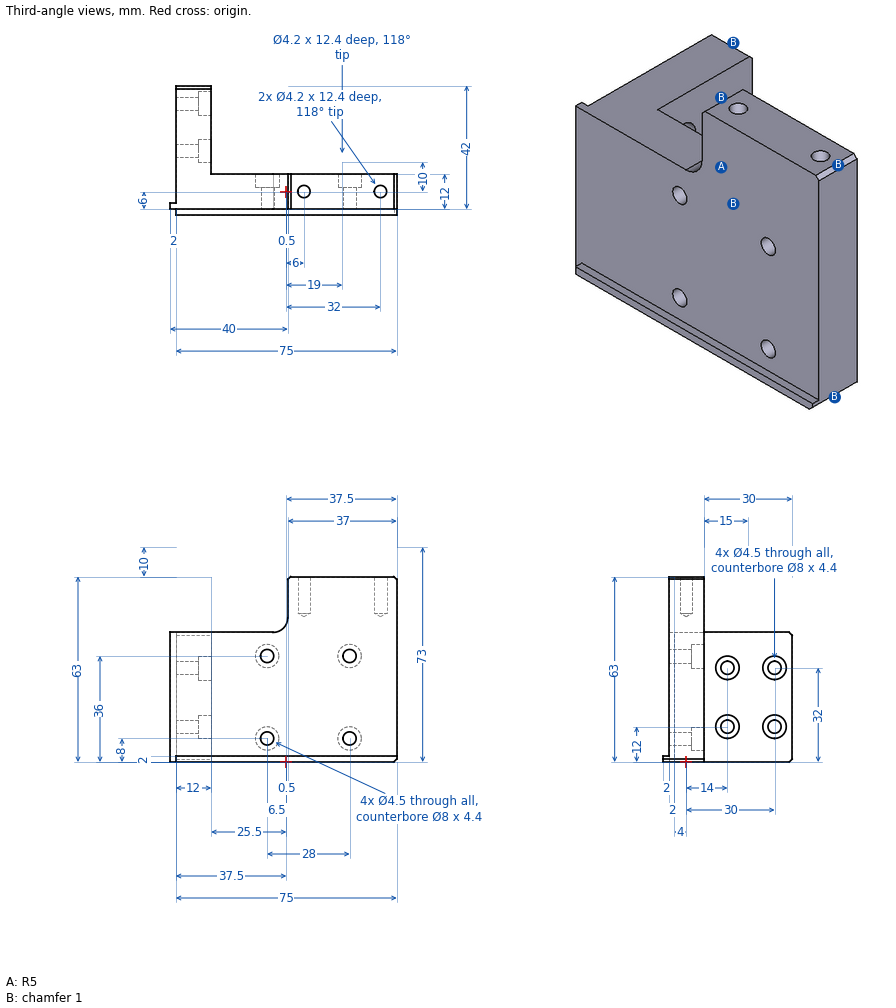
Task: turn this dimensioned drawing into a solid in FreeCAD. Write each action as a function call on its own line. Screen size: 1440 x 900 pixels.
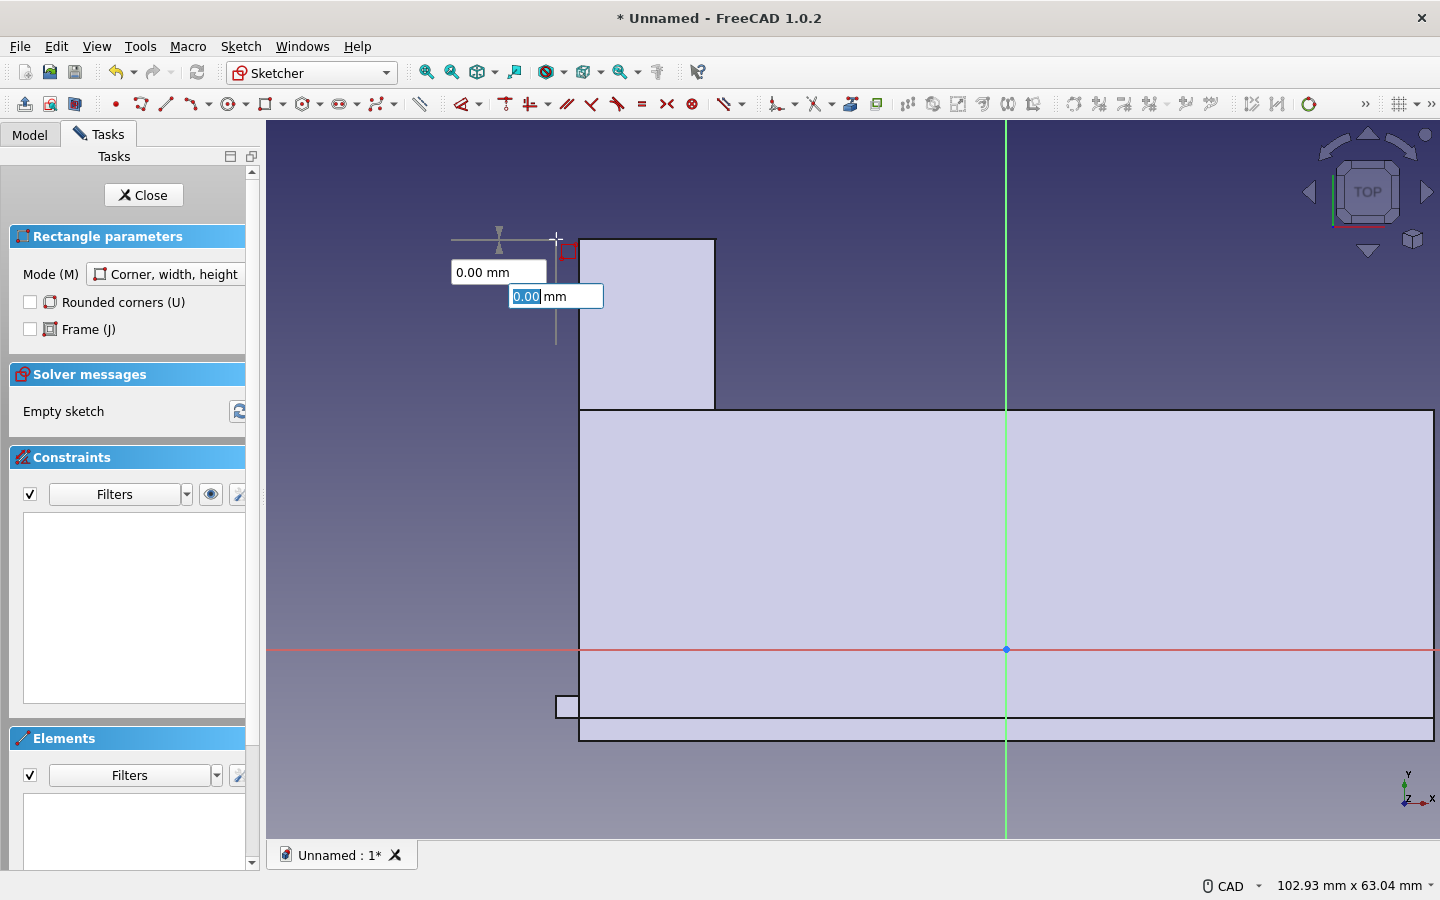
scroll(1012, 718, up, 6)
move(1011, 717)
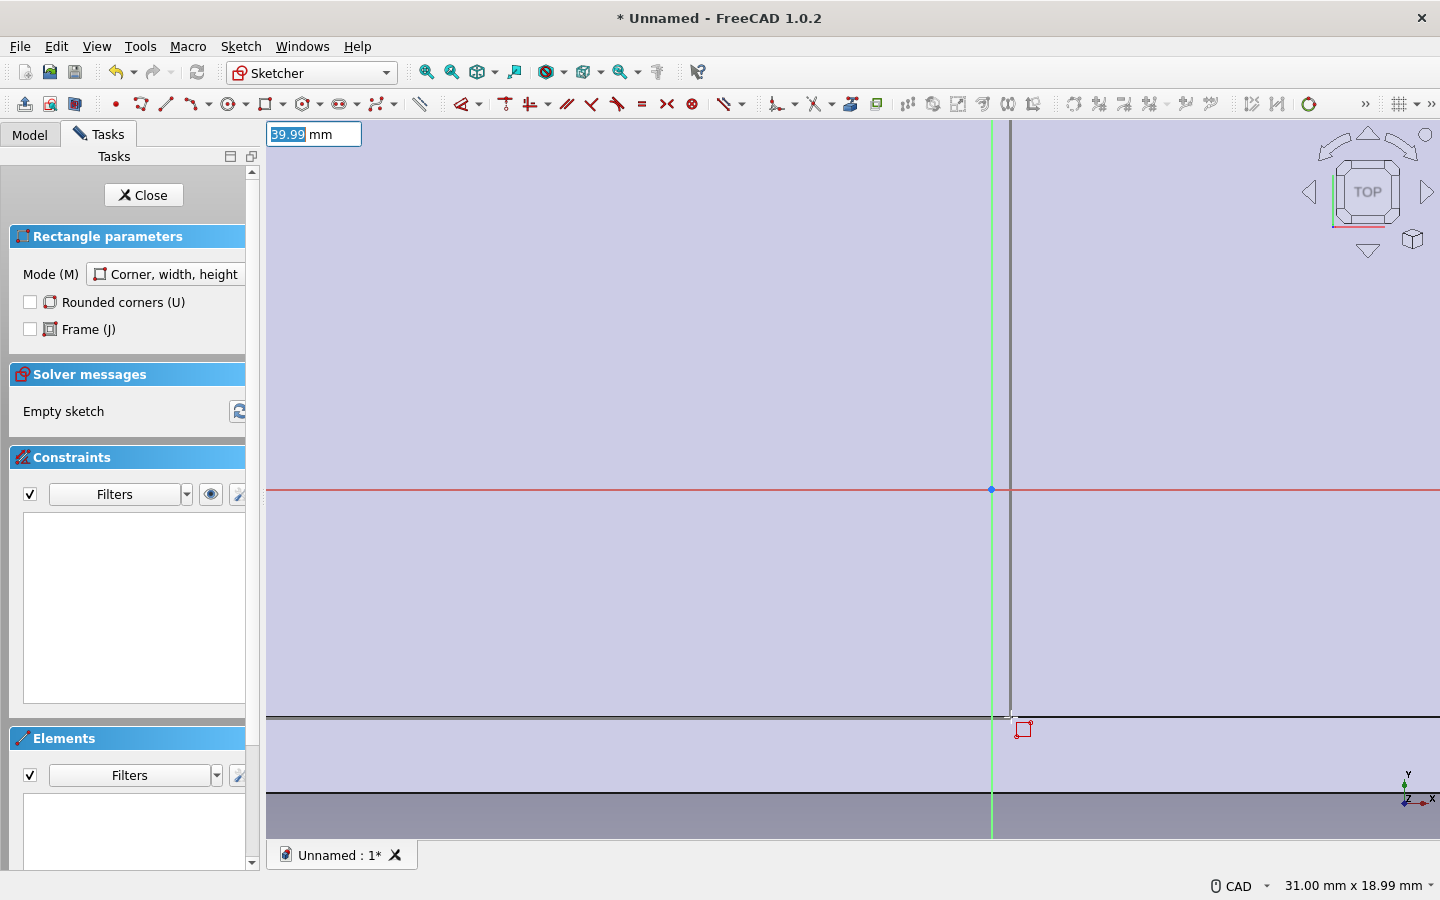
text(40)
key(Tab)
text(42)
key(Return)
key(Escape)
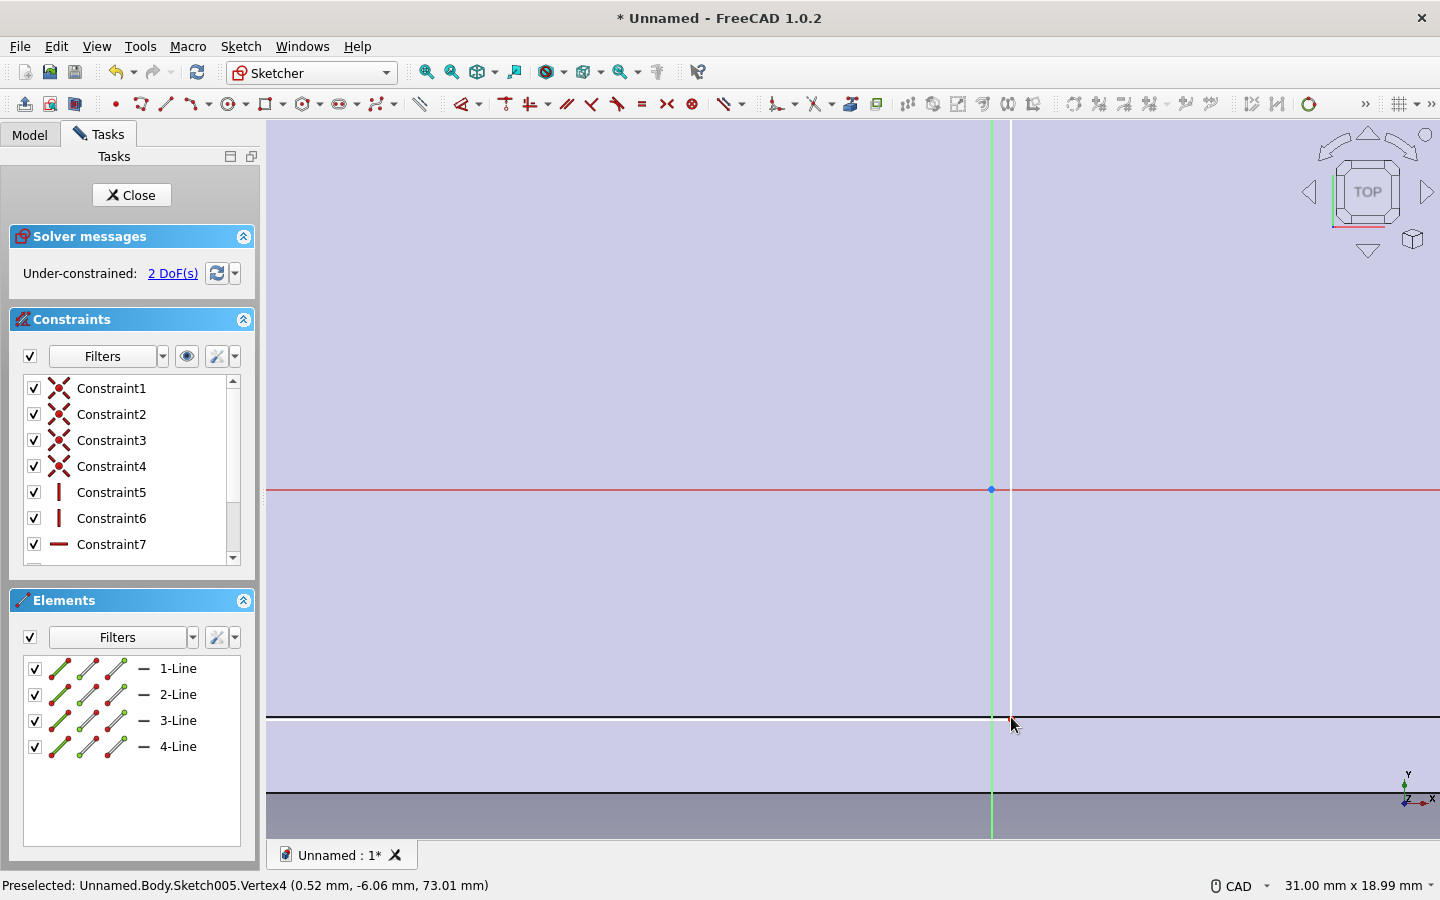
key(d)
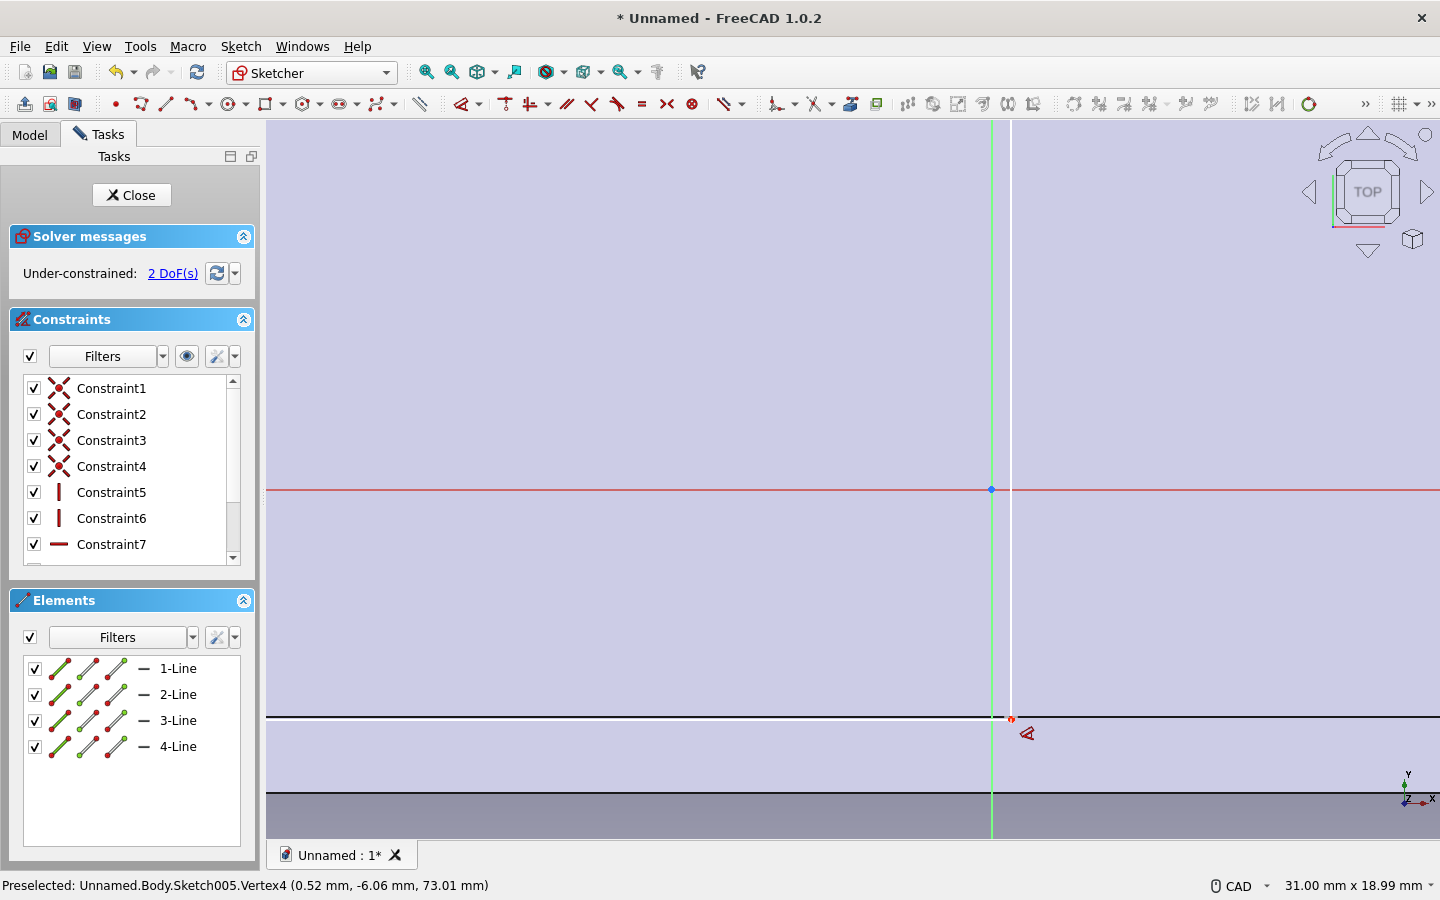
scroll(1013, 720, down, 6)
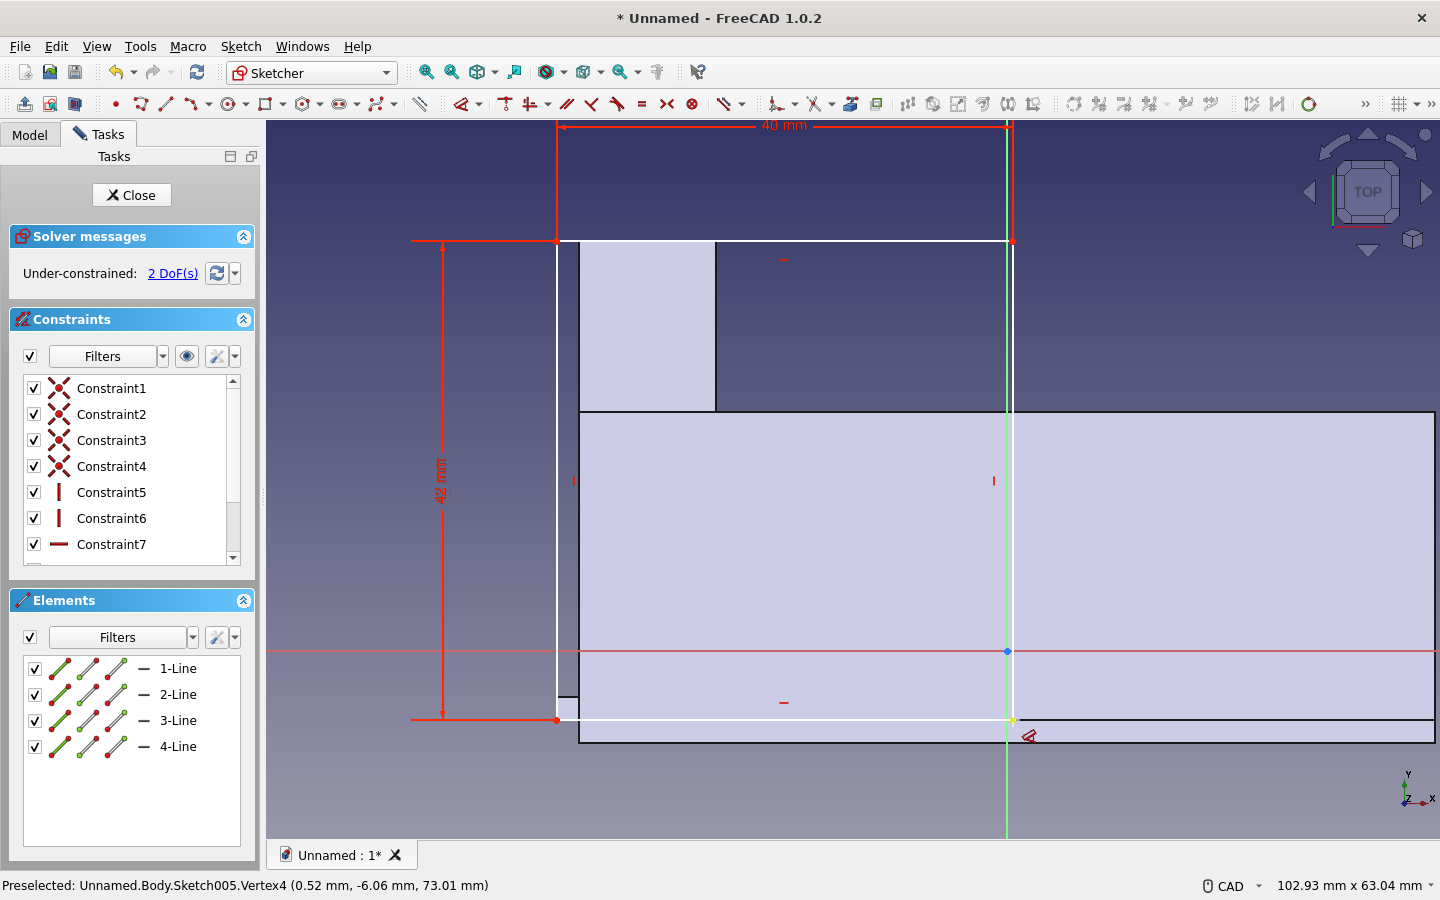
click(557, 720)
click(523, 686)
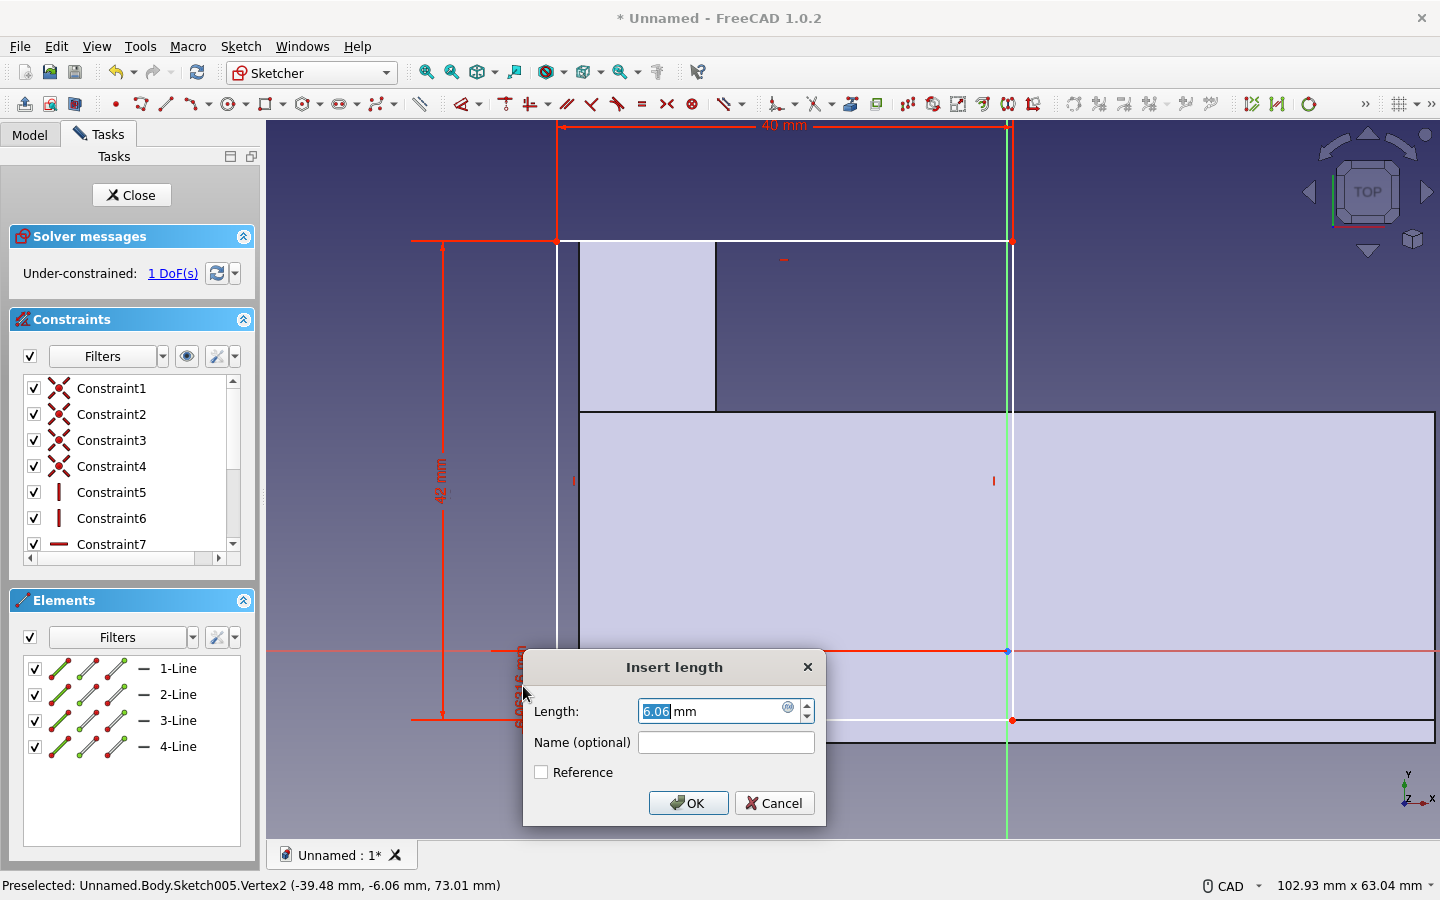
text(6)
key(Return)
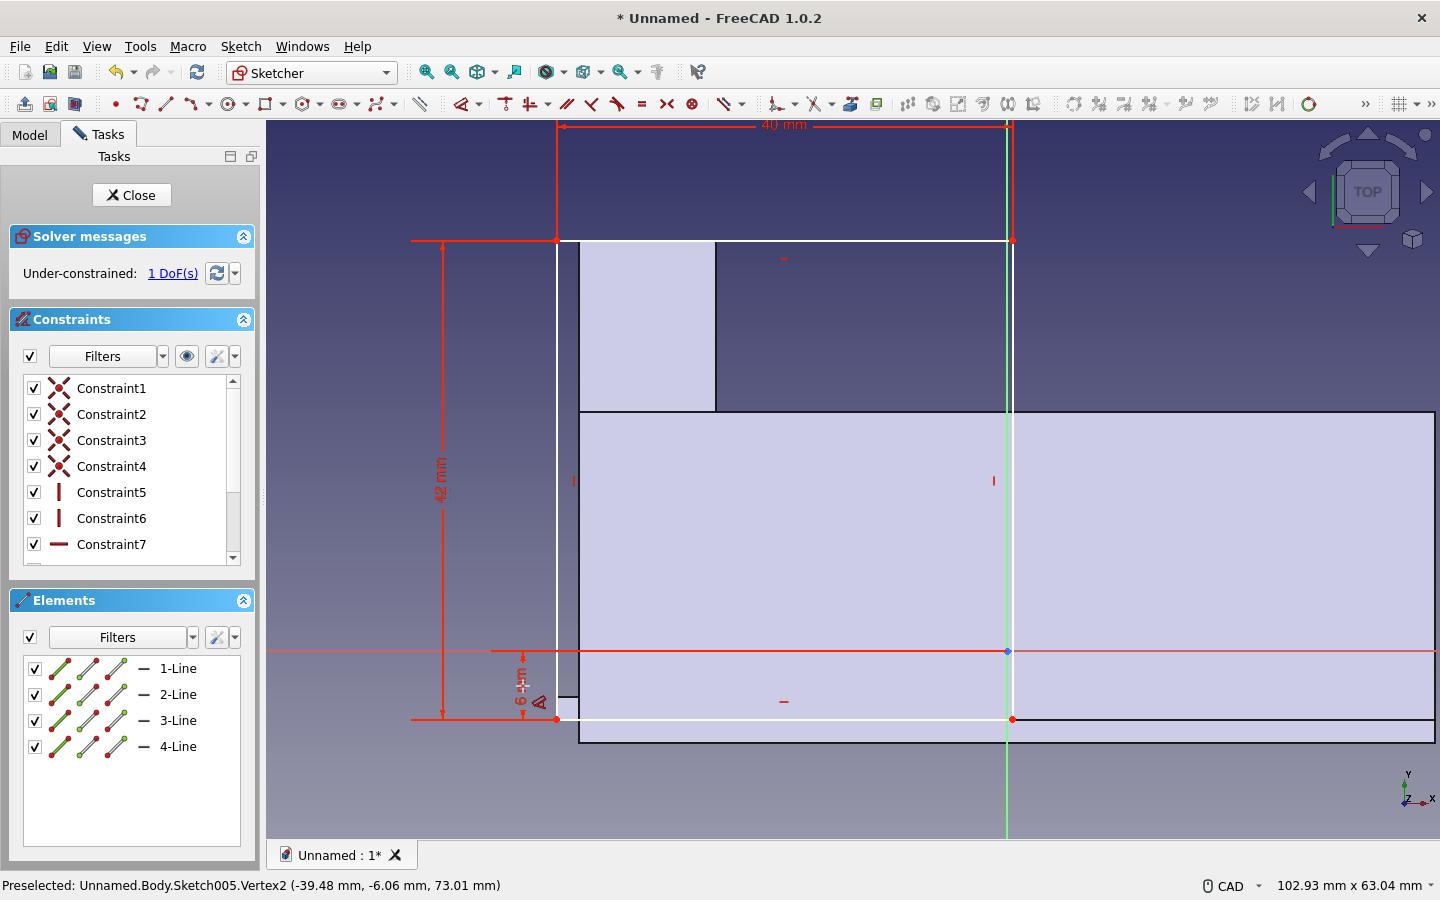
scroll(1013, 720, up, 10)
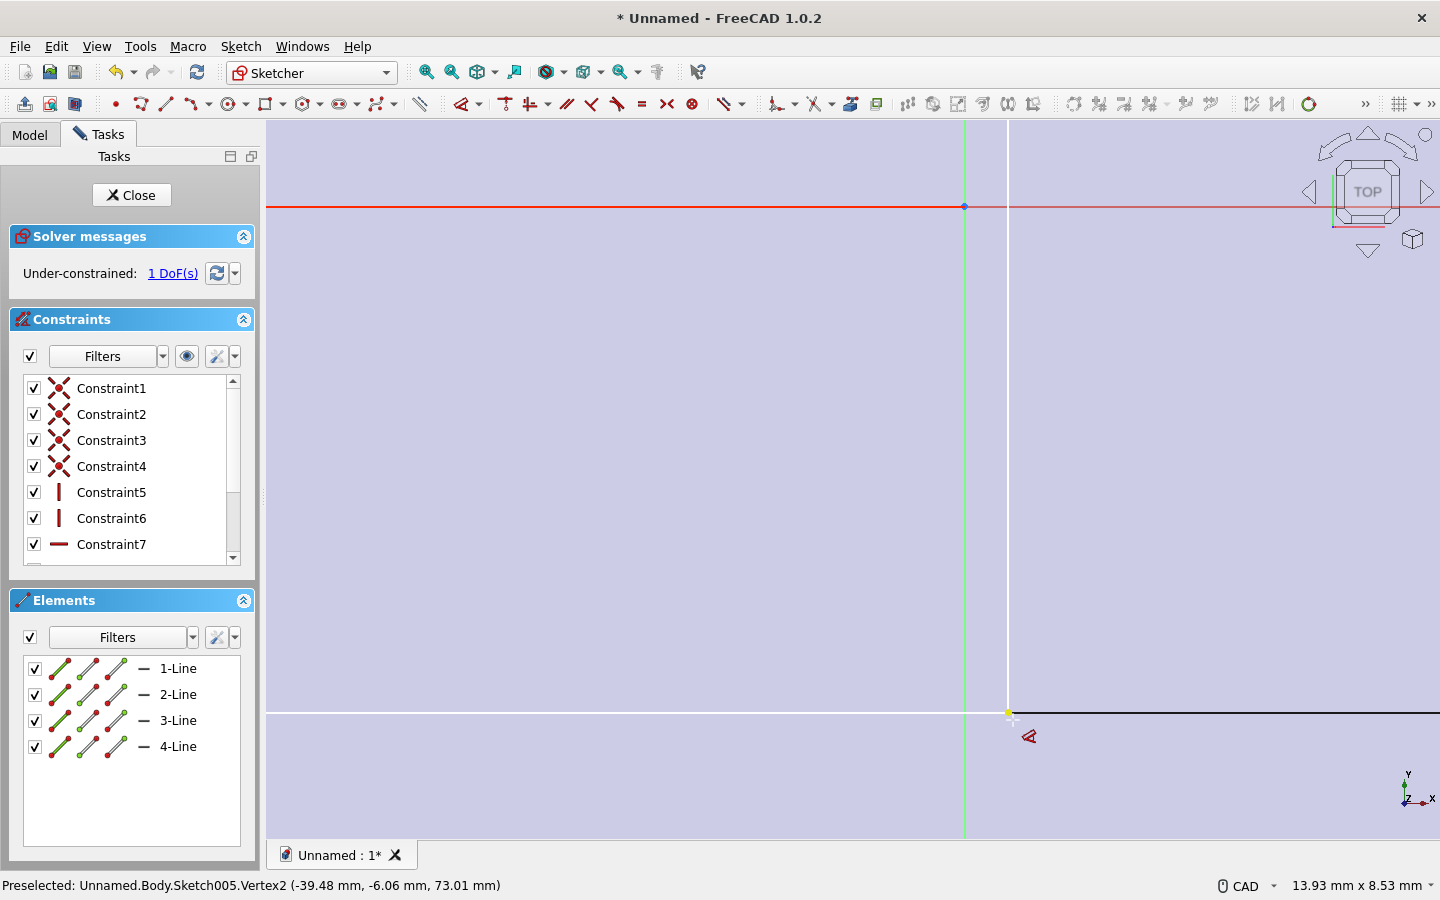
click(1008, 713)
click(987, 747)